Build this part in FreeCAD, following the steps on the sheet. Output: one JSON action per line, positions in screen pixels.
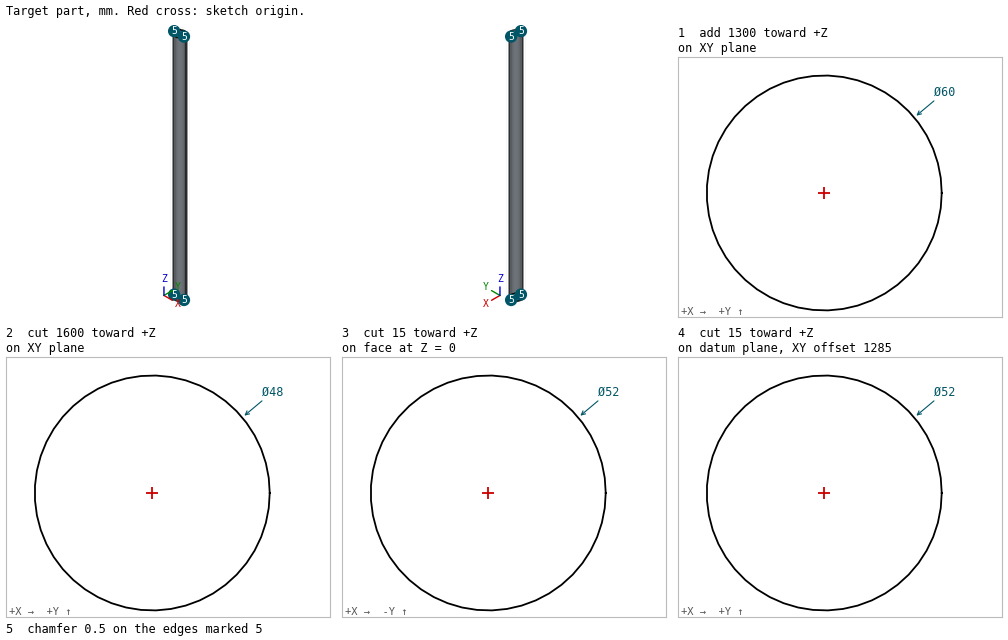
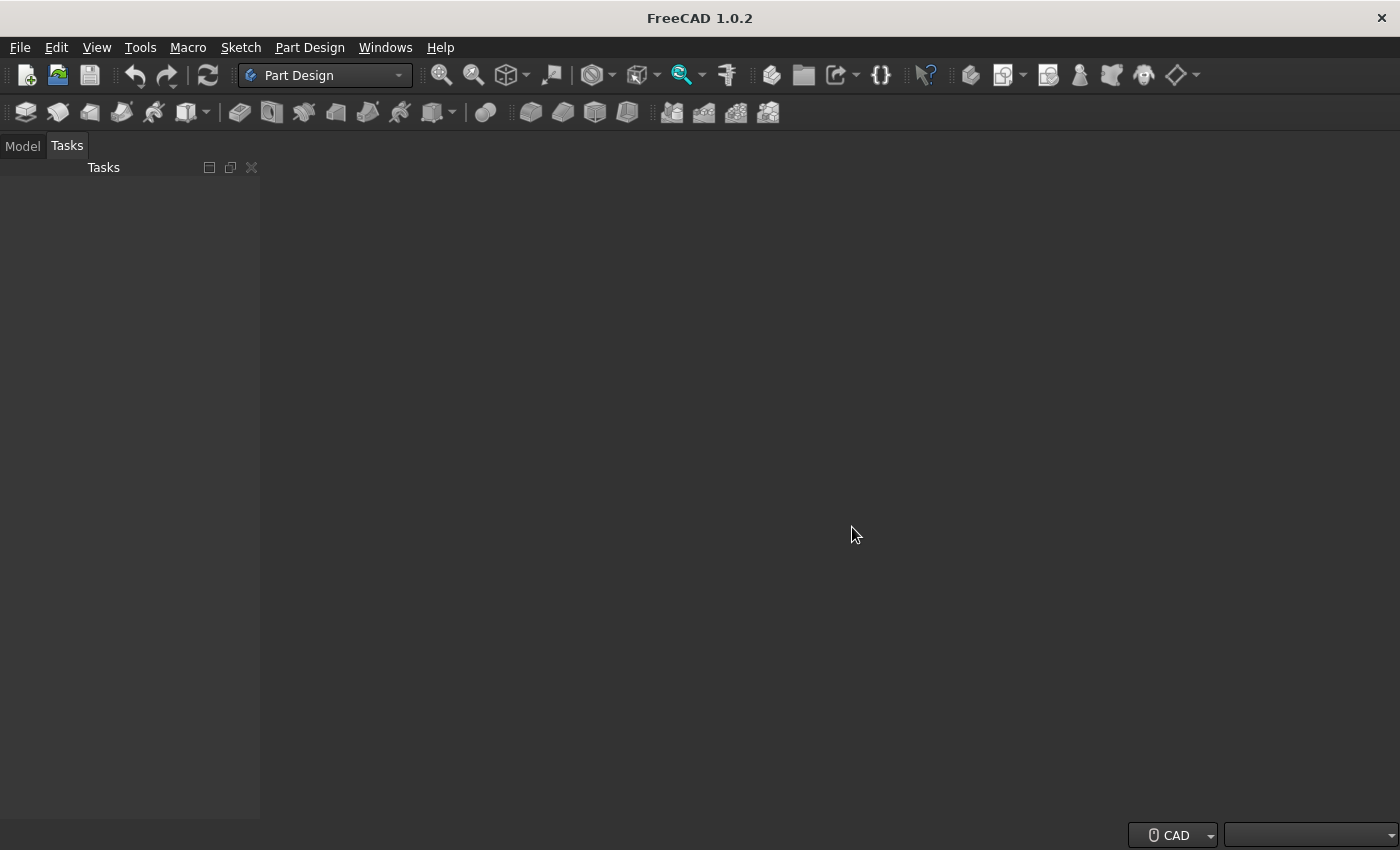
{"action": "left_click", "coordinate": [26, 76]}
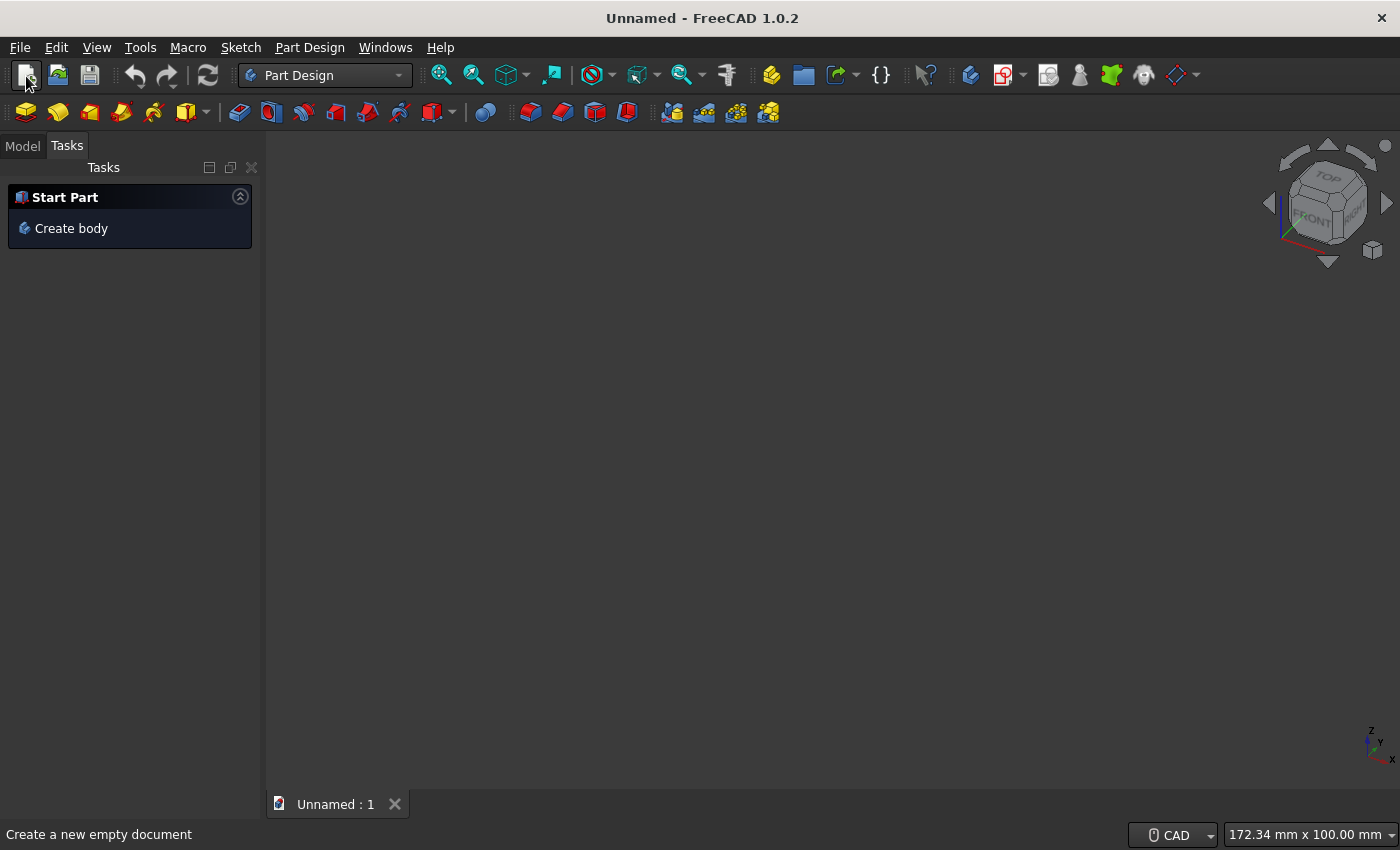
{"action": "left_click", "coordinate": [1004, 76]}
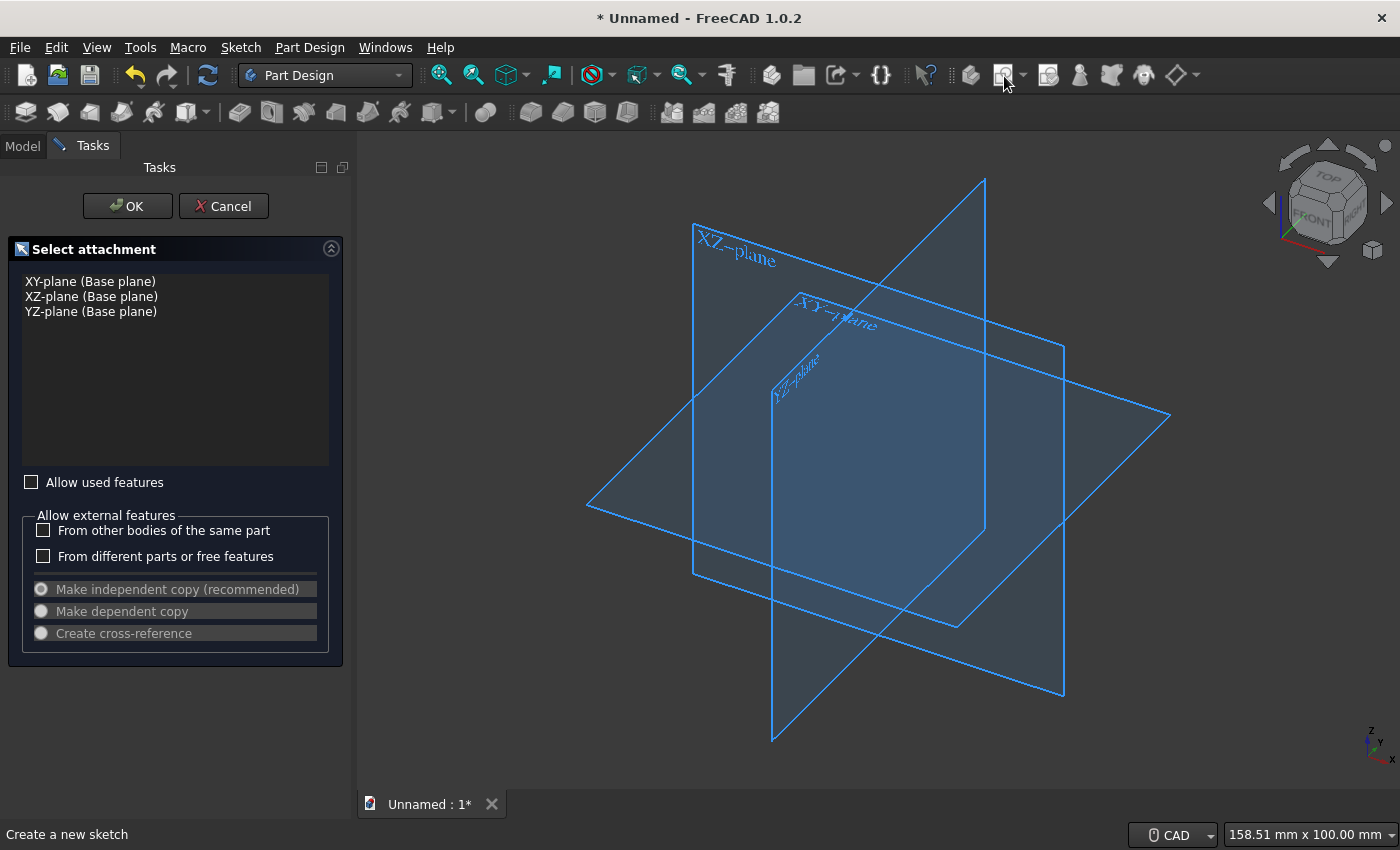
{"action": "left_click", "coordinate": [82, 282]}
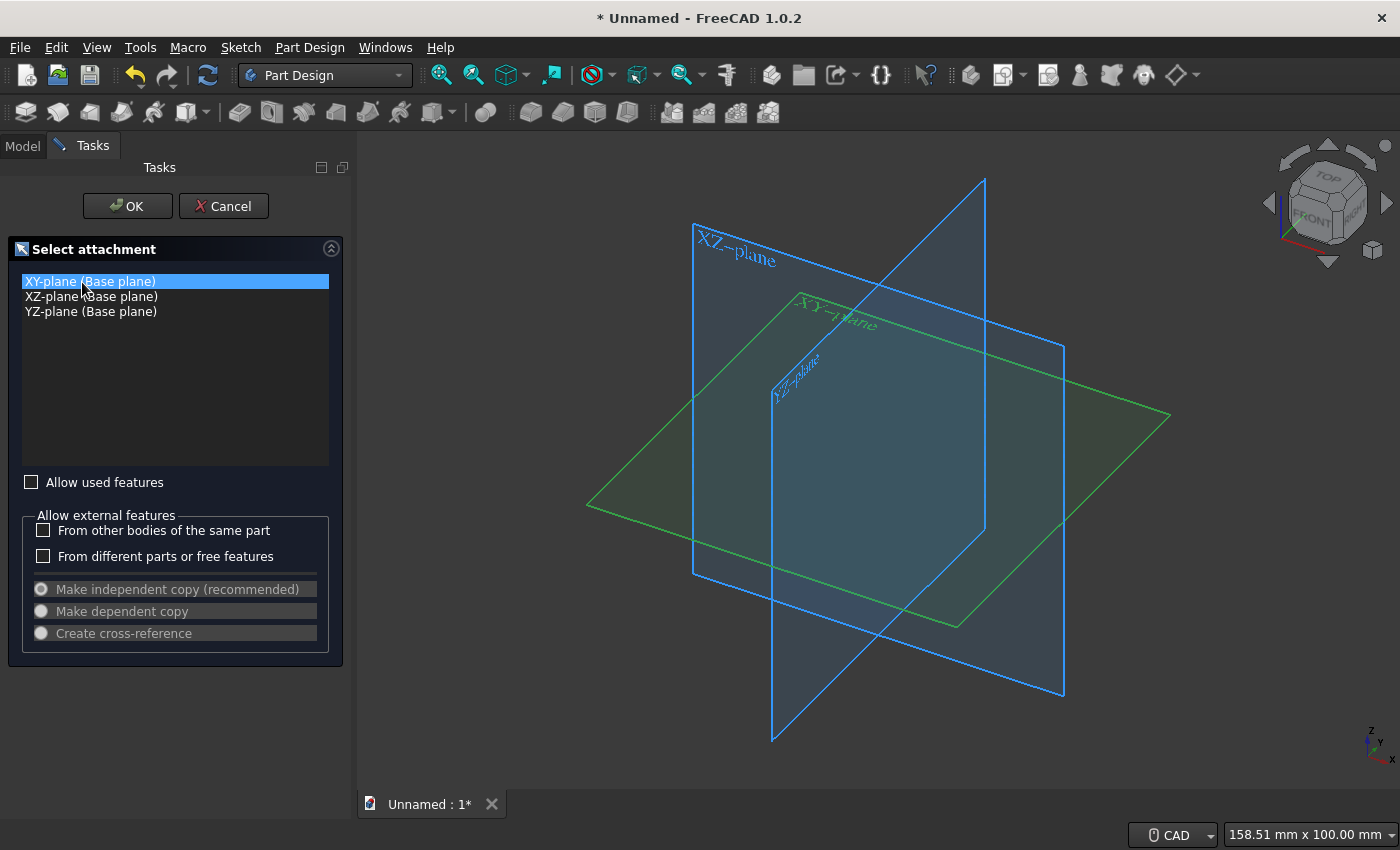
{"action": "left_click", "coordinate": [128, 206]}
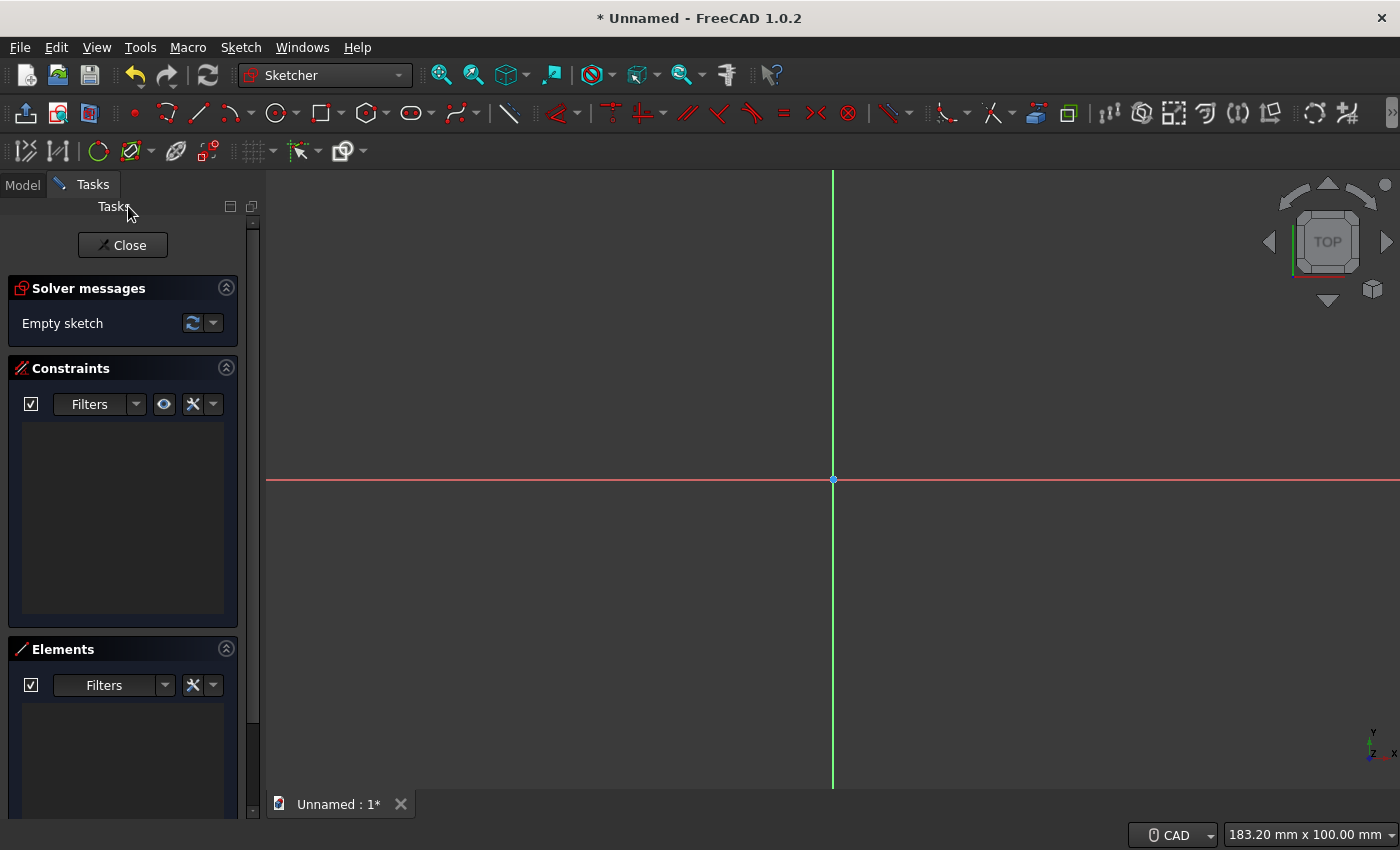
{"action": "left_click", "coordinate": [276, 114]}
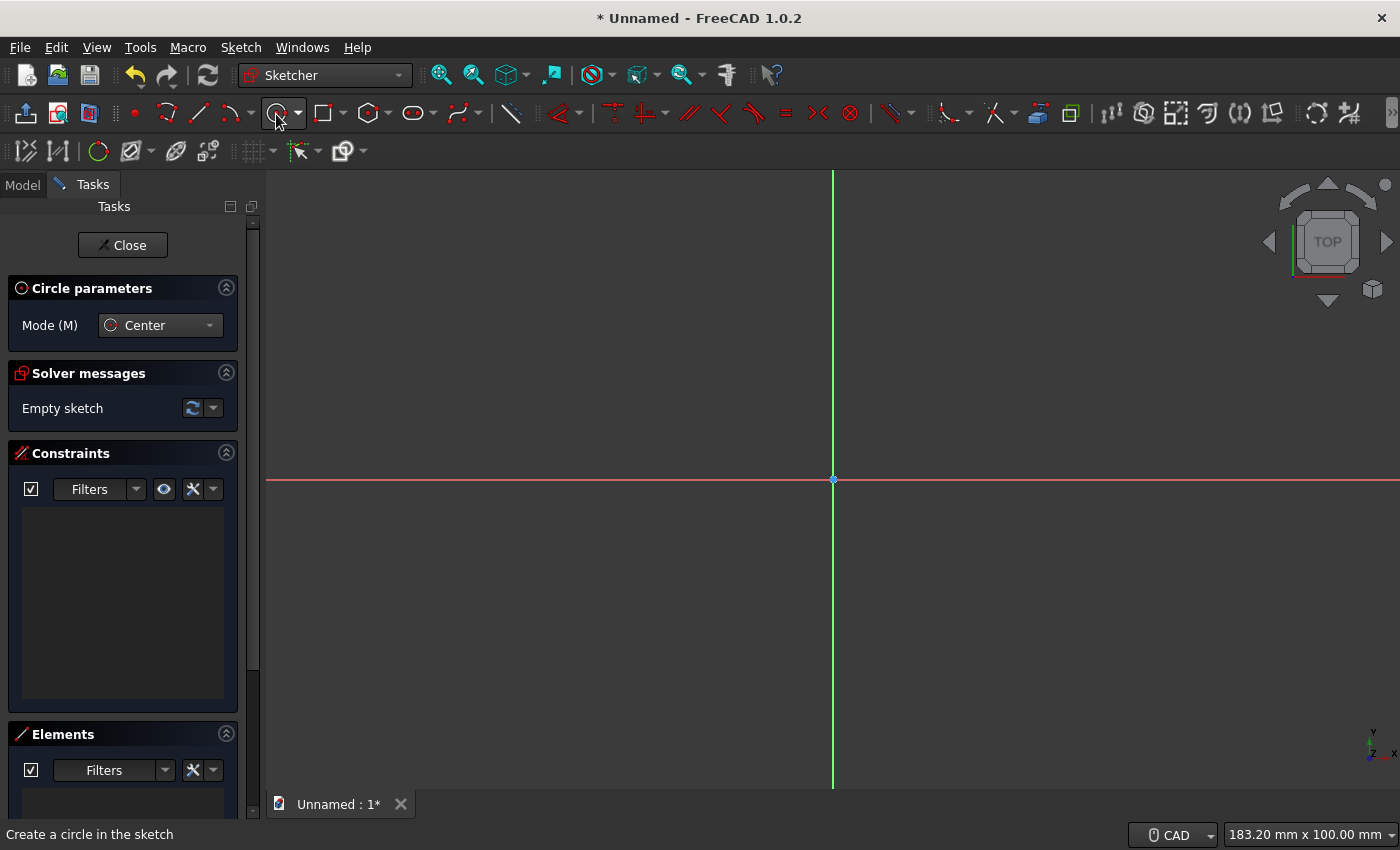
{"action": "left_click", "coordinate": [833, 480]}
{"action": "mouse_move", "coordinate": [964, 348]}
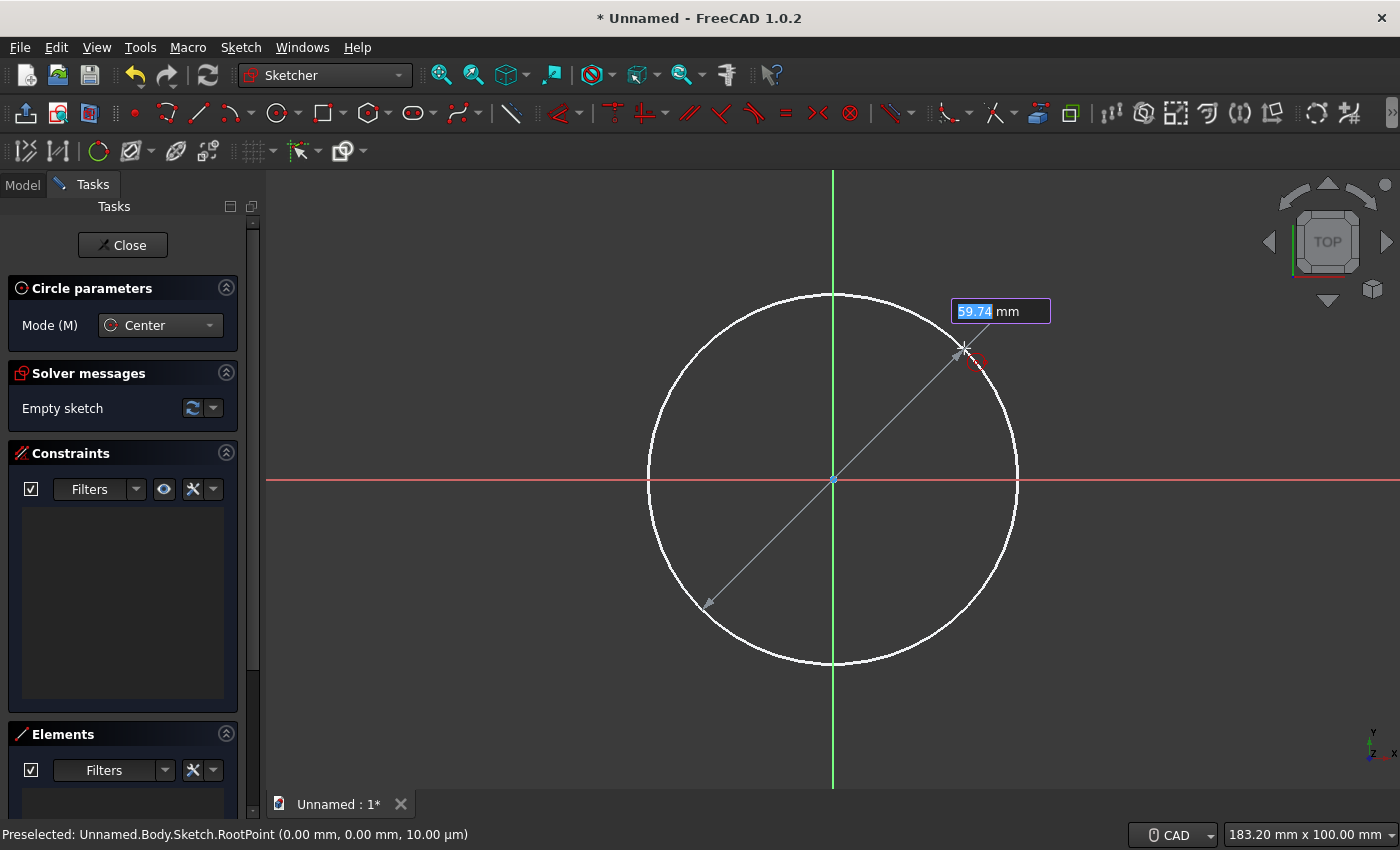
{"action": "type", "text": "60"}
{"action": "key", "text": "Return"}
{"action": "key", "text": "Escape"}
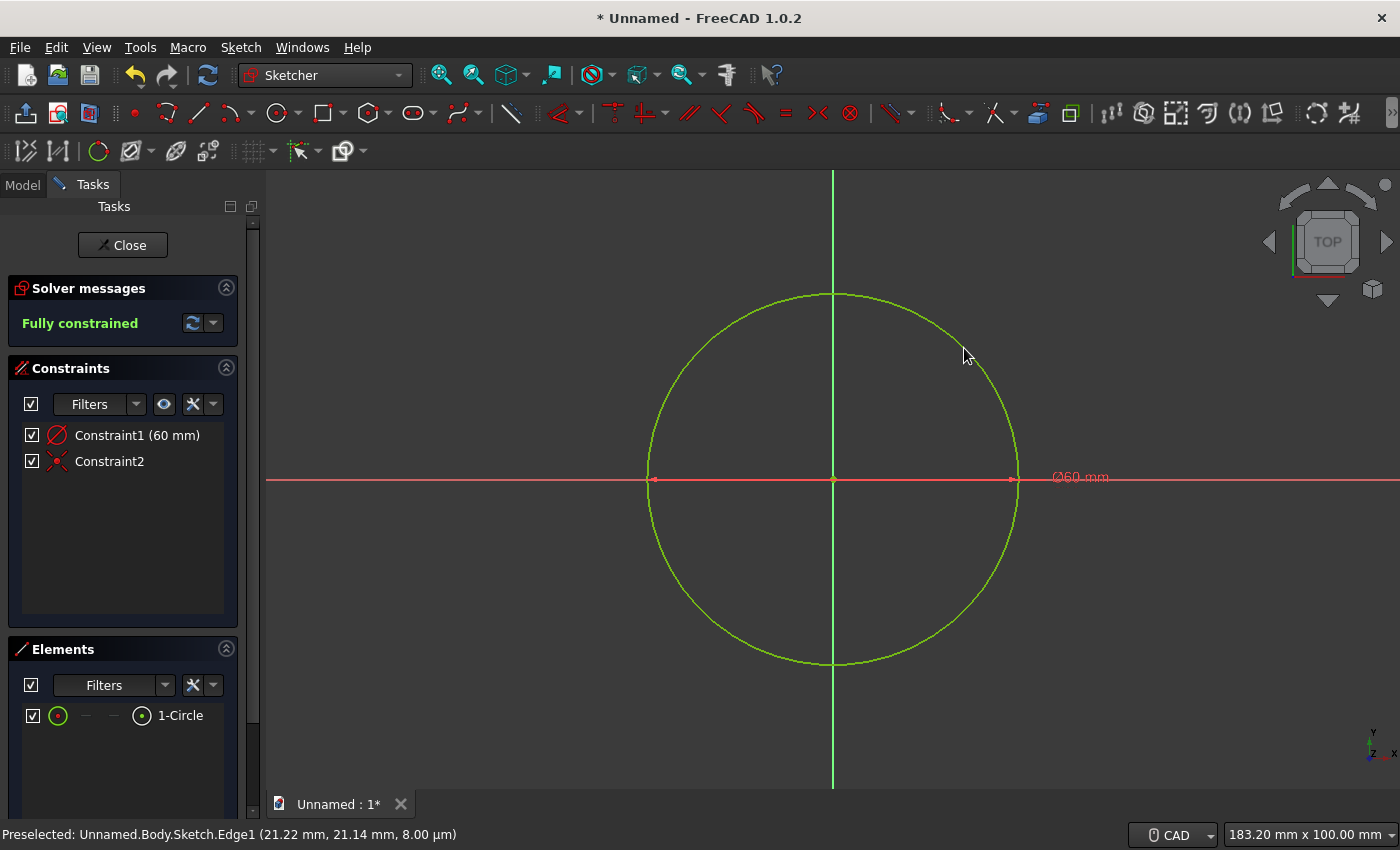
{"action": "left_click", "coordinate": [123, 245]}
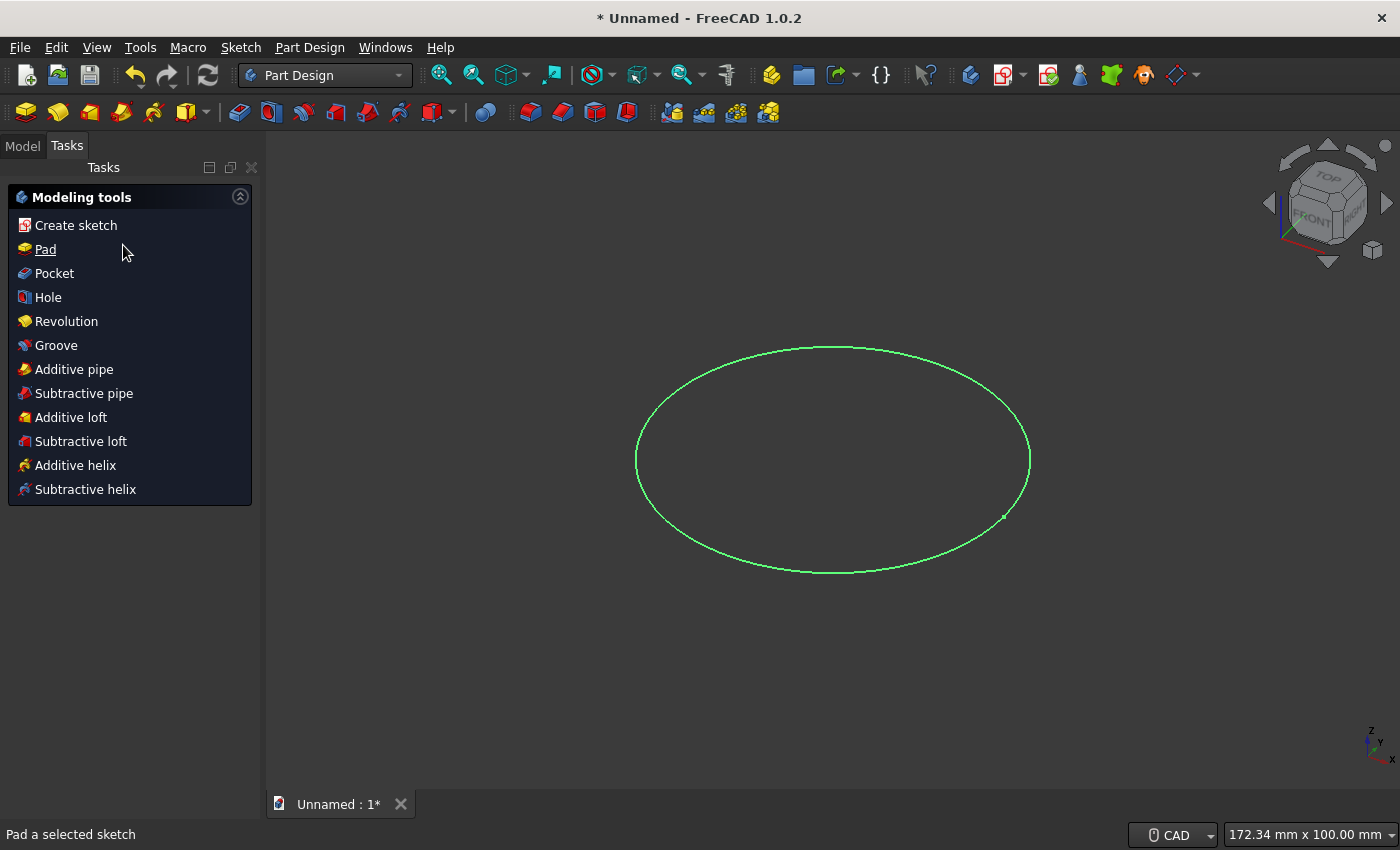
{"action": "left_click", "coordinate": [26, 112]}